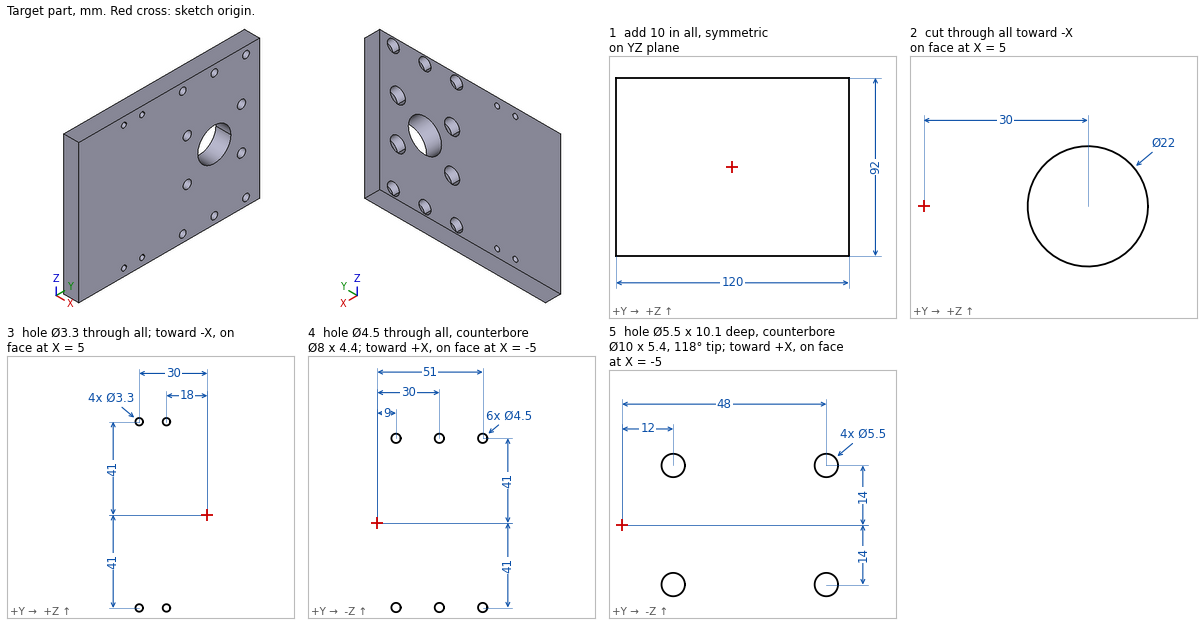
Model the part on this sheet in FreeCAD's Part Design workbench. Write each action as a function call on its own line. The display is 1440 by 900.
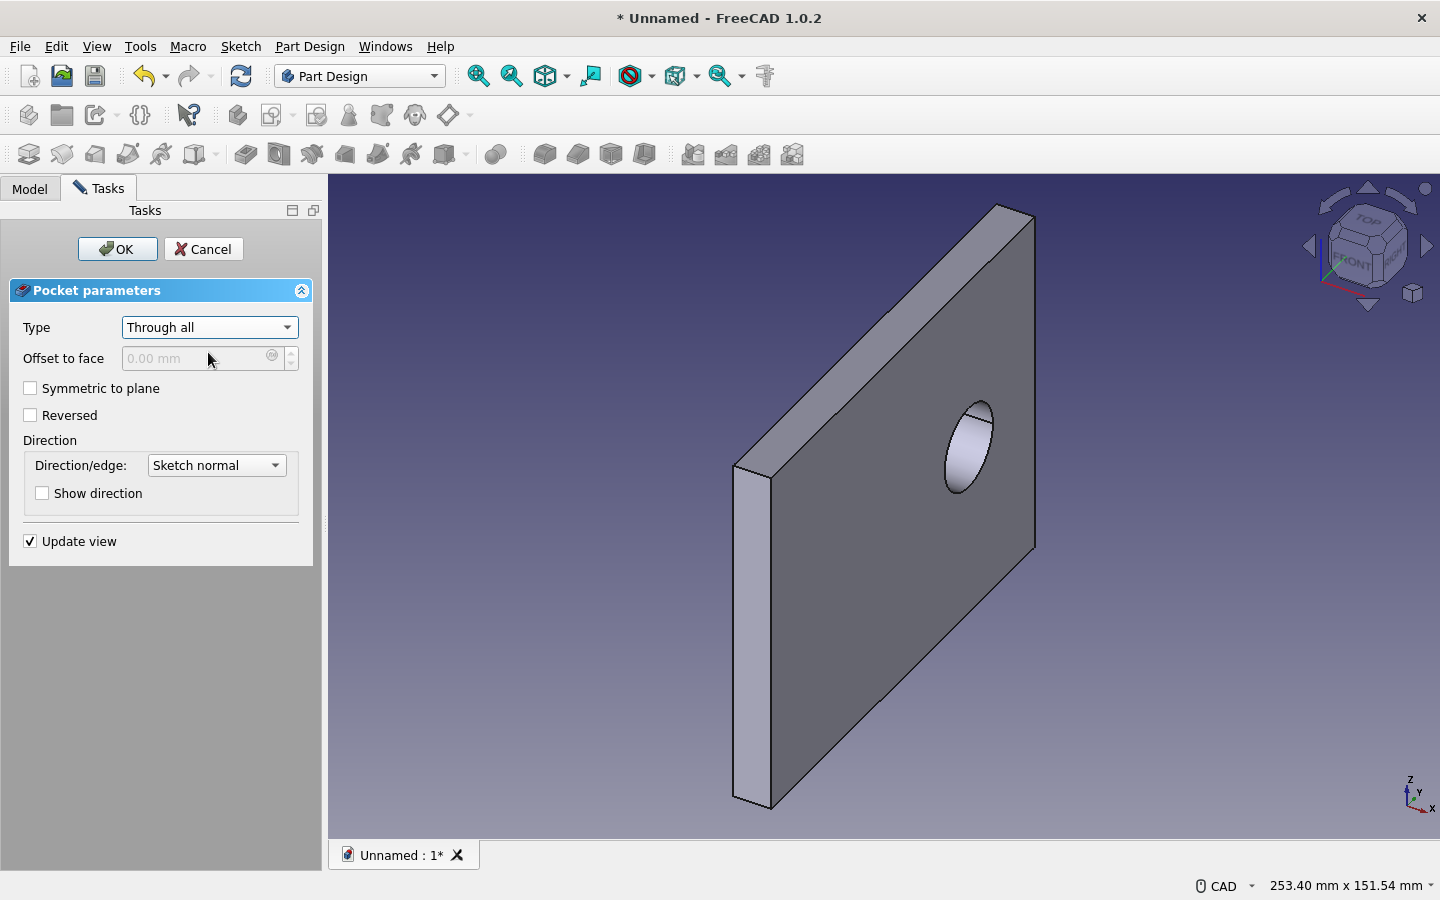
click(118, 249)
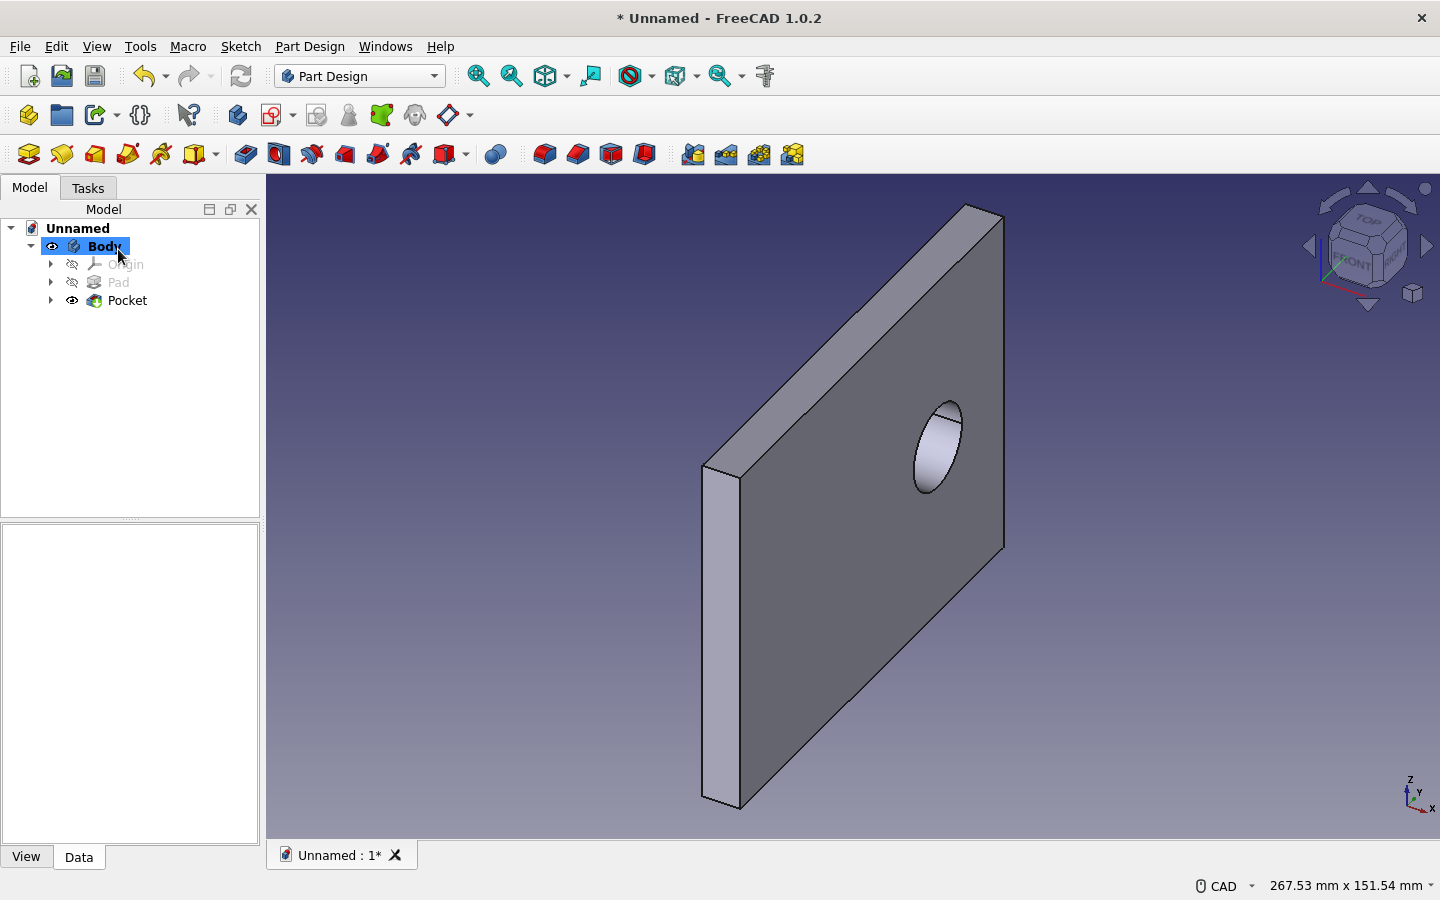
click(834, 549)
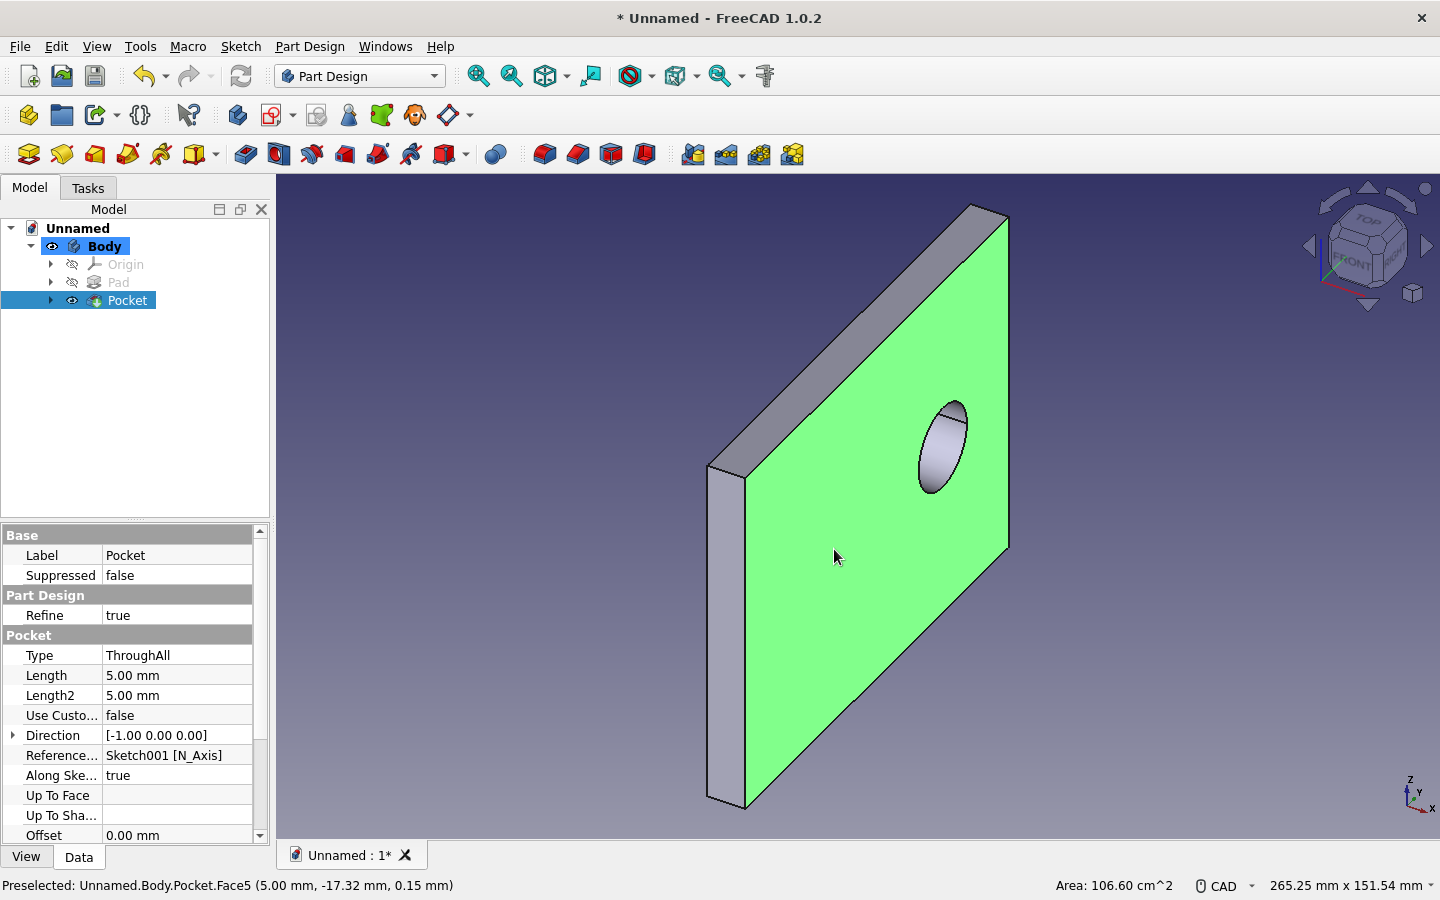
click(270, 116)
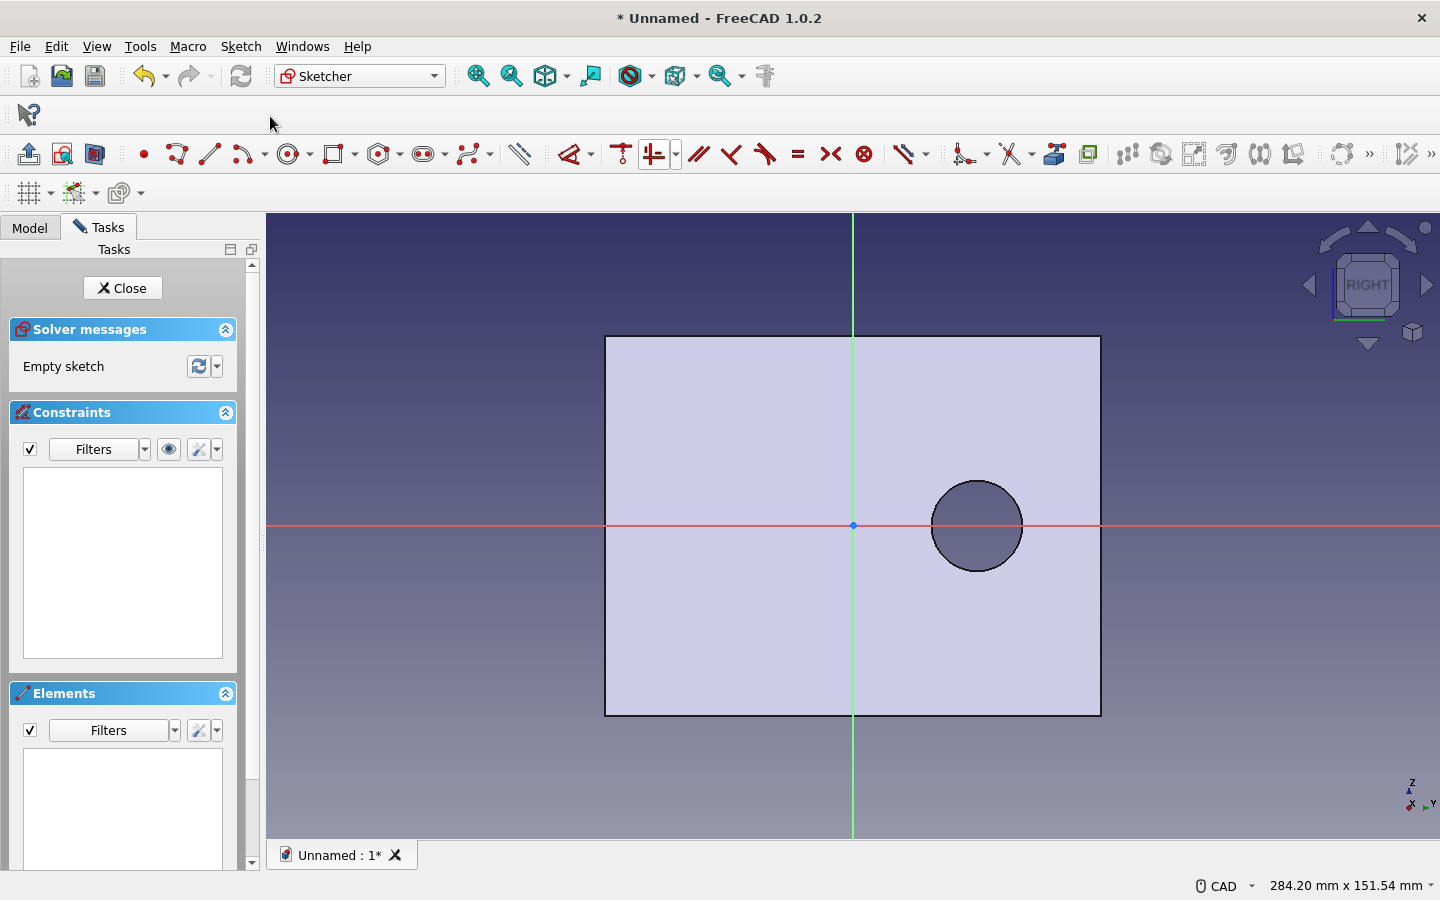
key(g)
key(c)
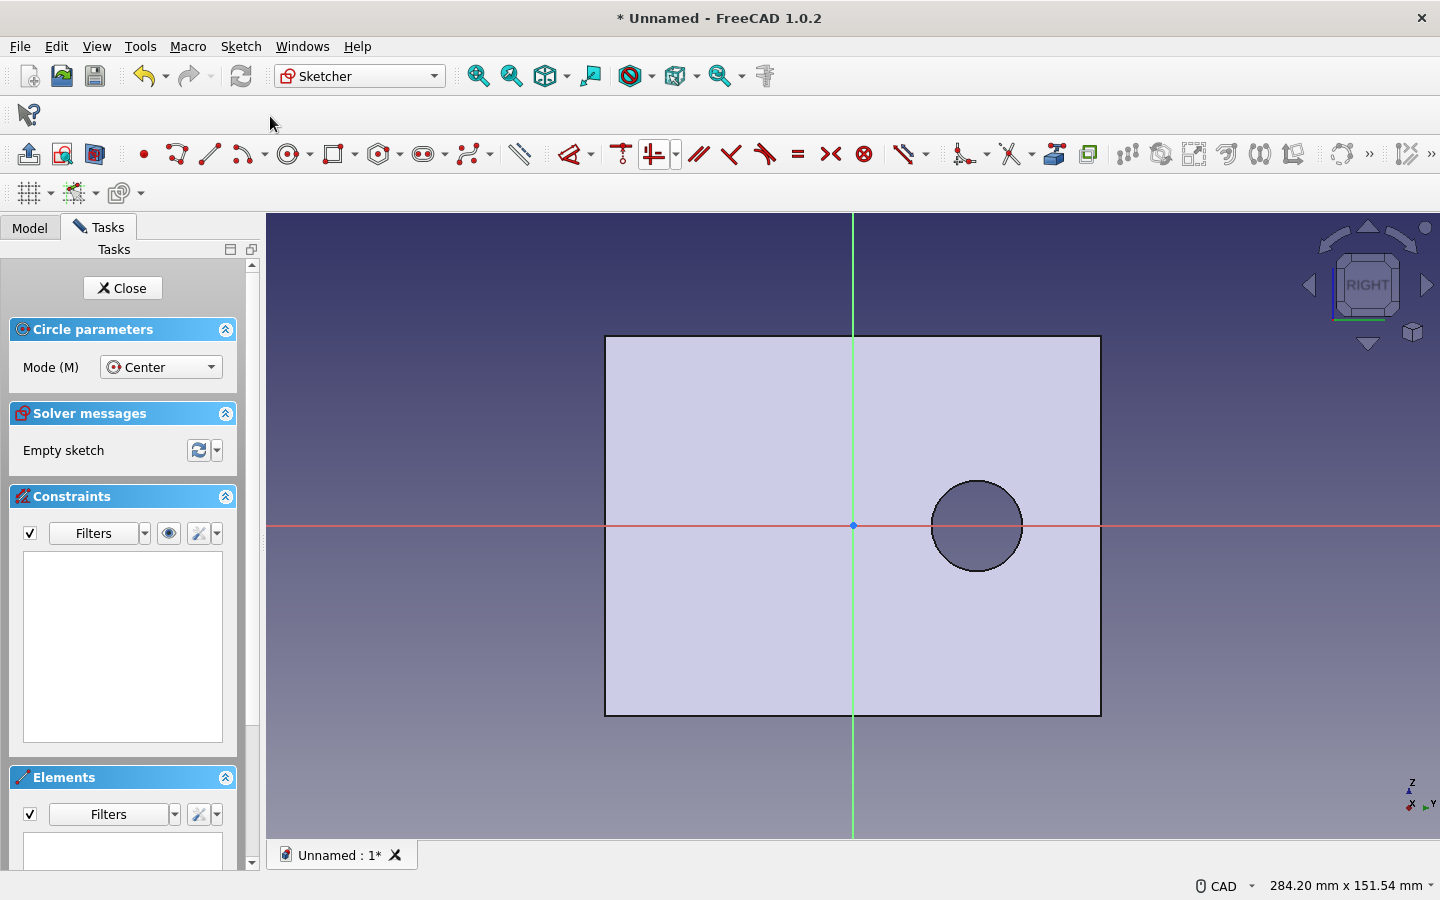
scroll(729, 357, up, 7)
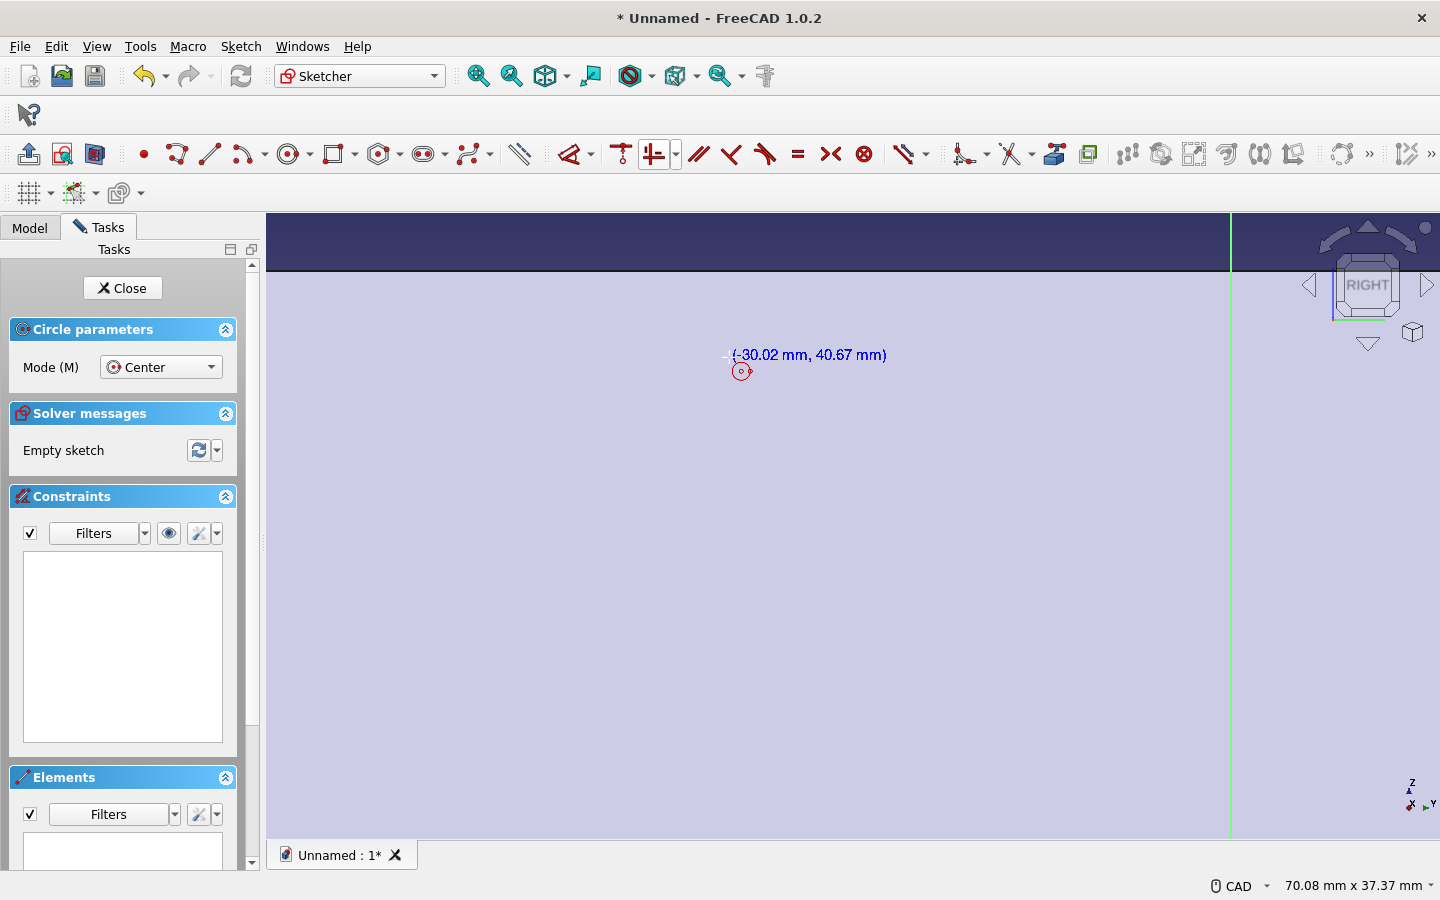
scroll(706, 304, down, 6)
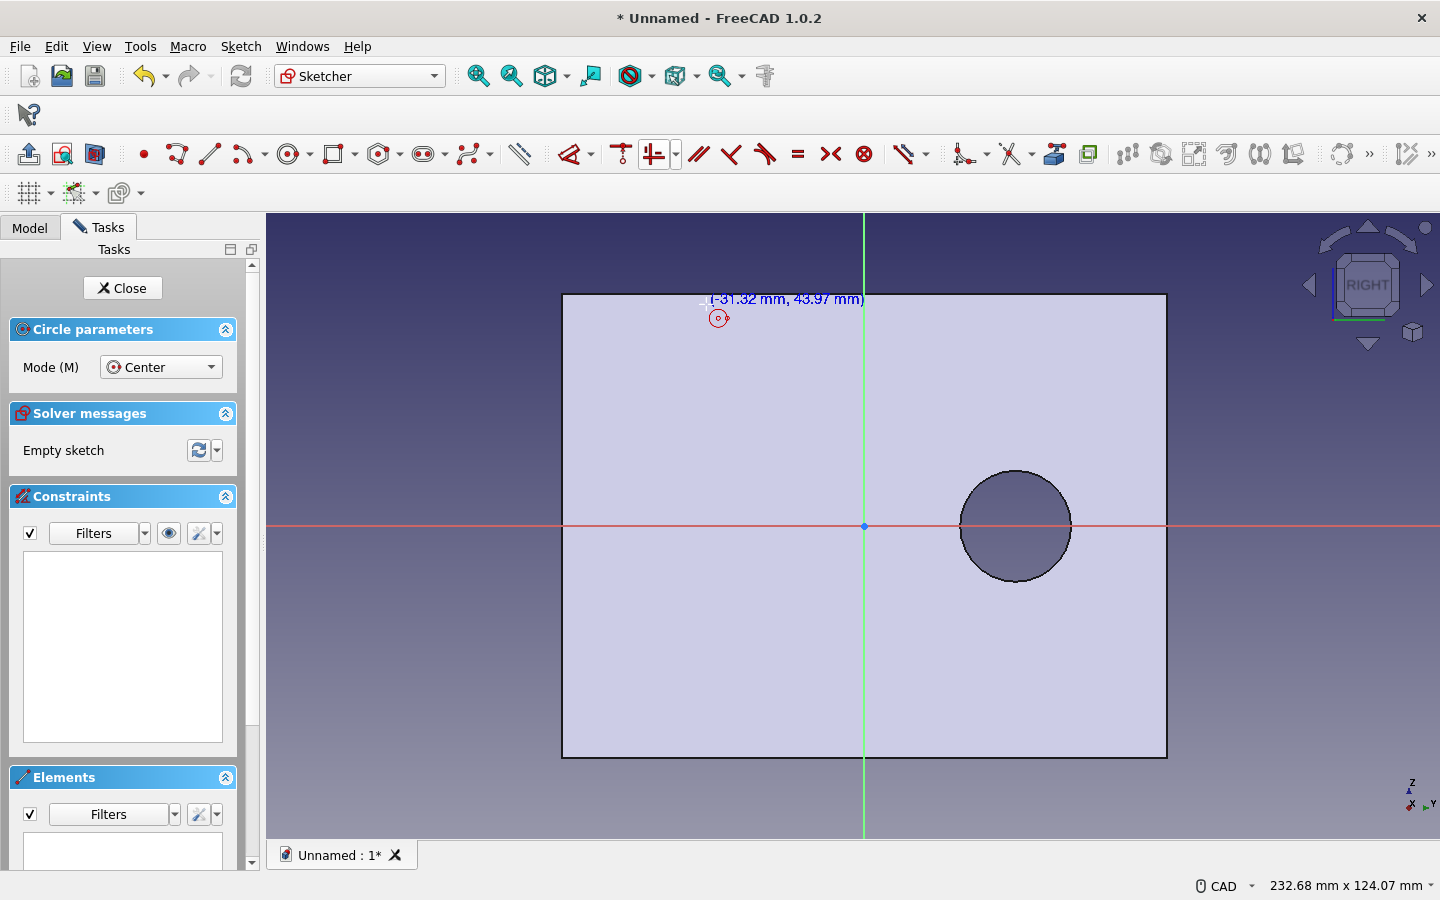
click(713, 319)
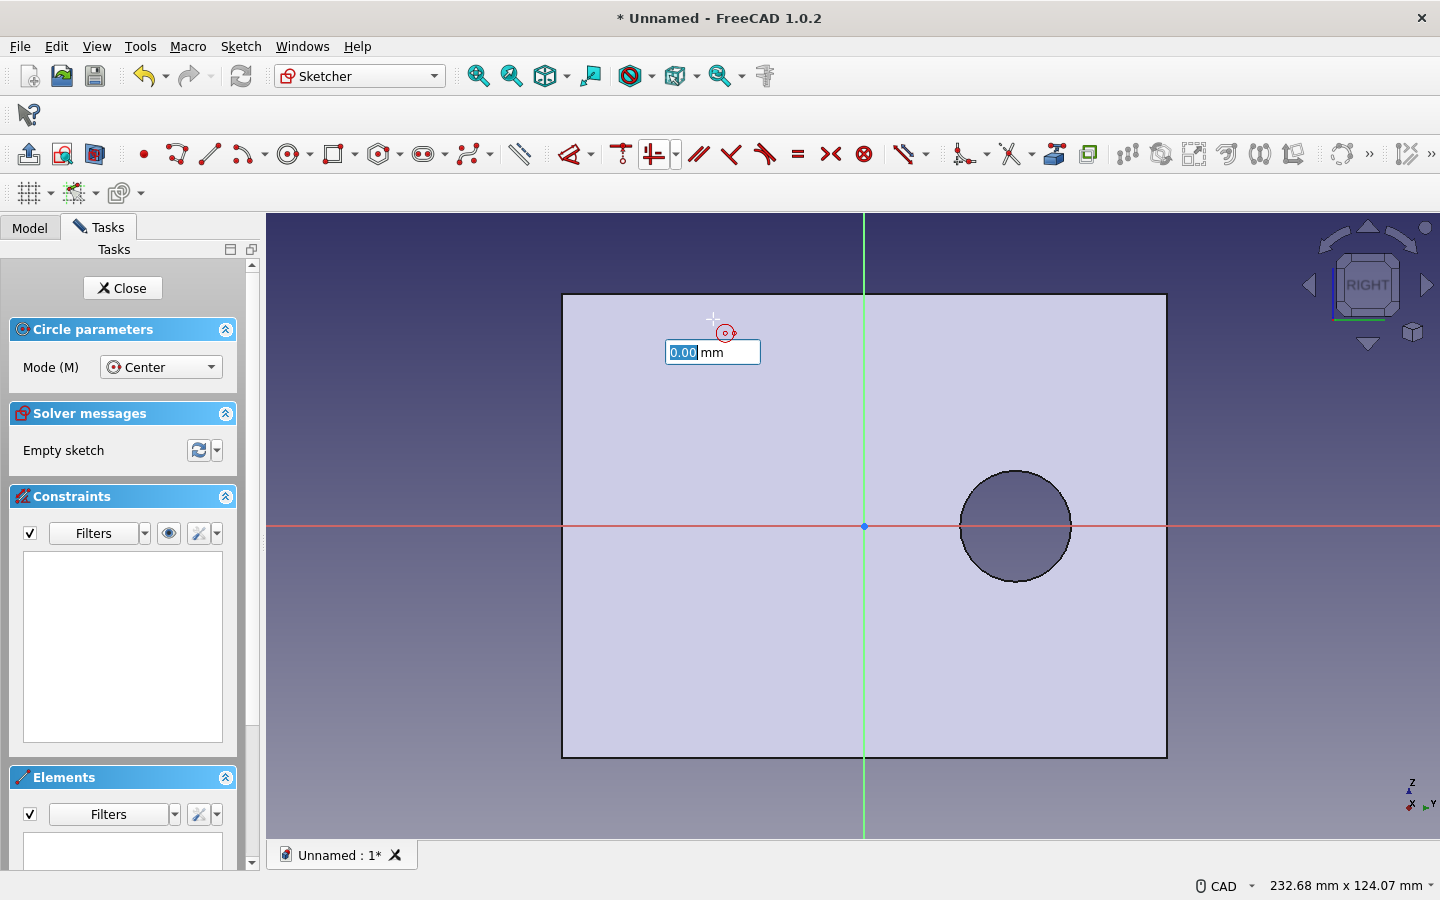
scroll(719, 314, up, 4)